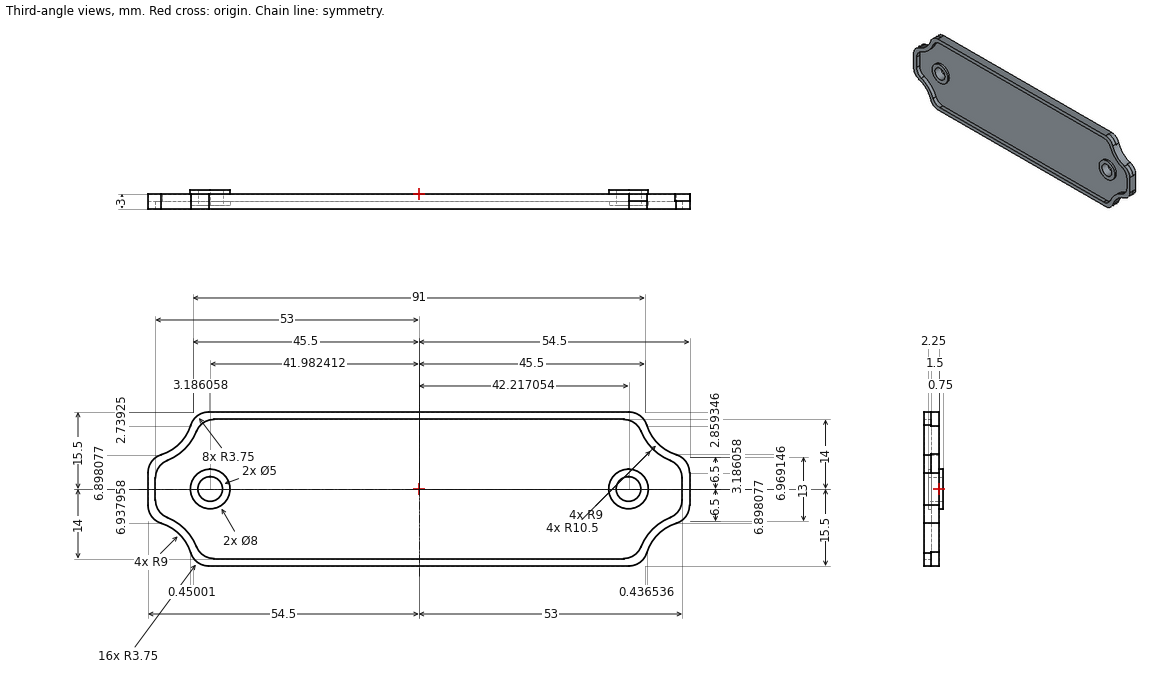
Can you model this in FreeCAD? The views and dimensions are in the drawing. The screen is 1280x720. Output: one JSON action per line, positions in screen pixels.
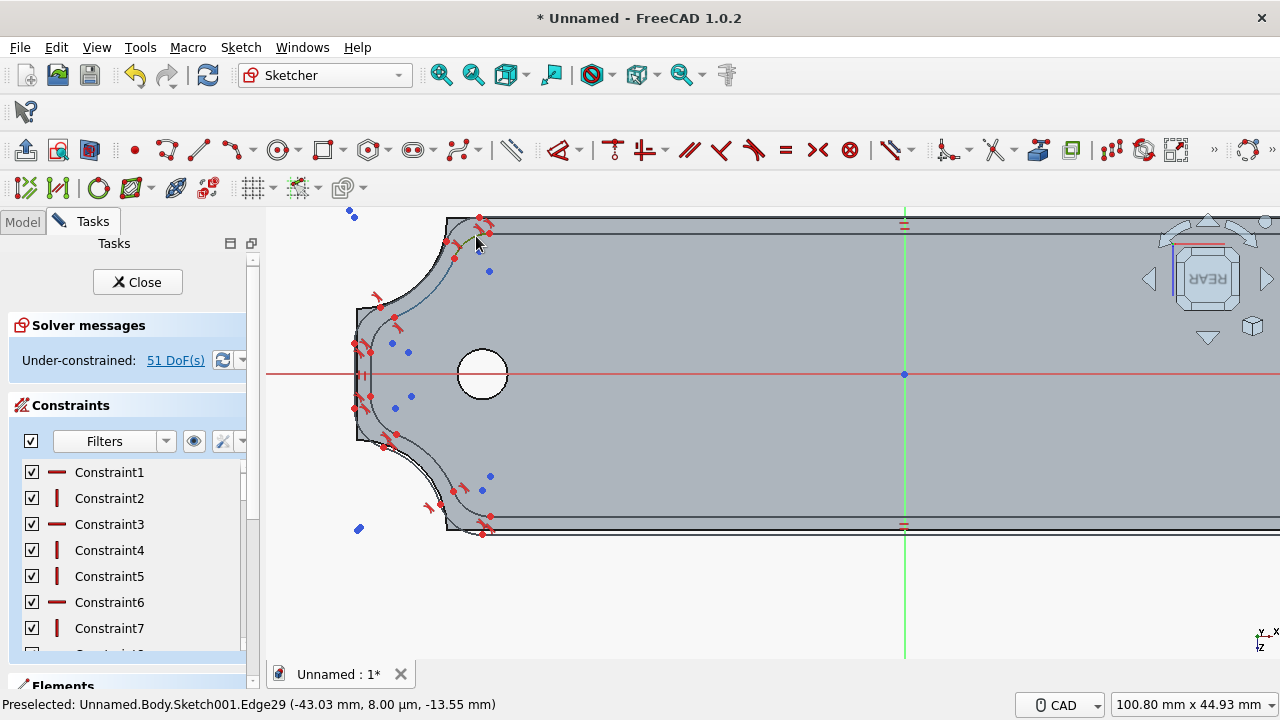
{"action": "left_click", "coordinate": [754, 150]}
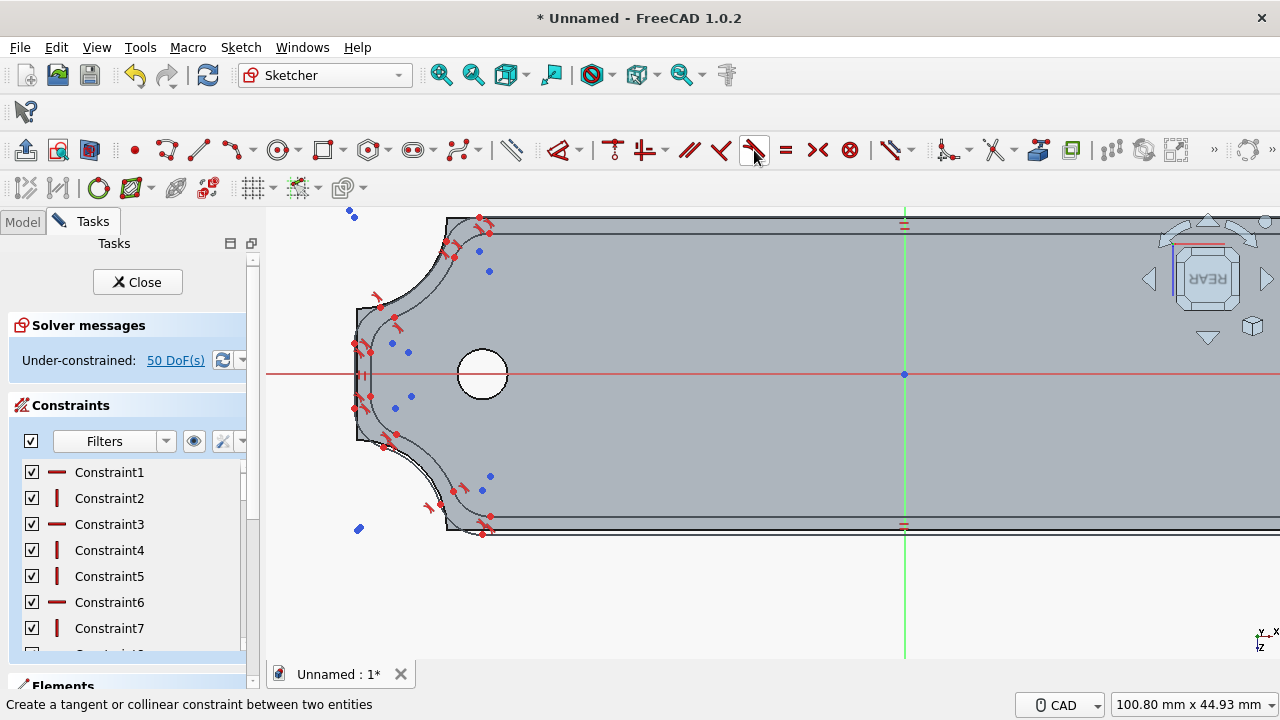
{"action": "scroll", "coordinate": [461, 504], "scroll_direction": "down", "scroll_amount": 3}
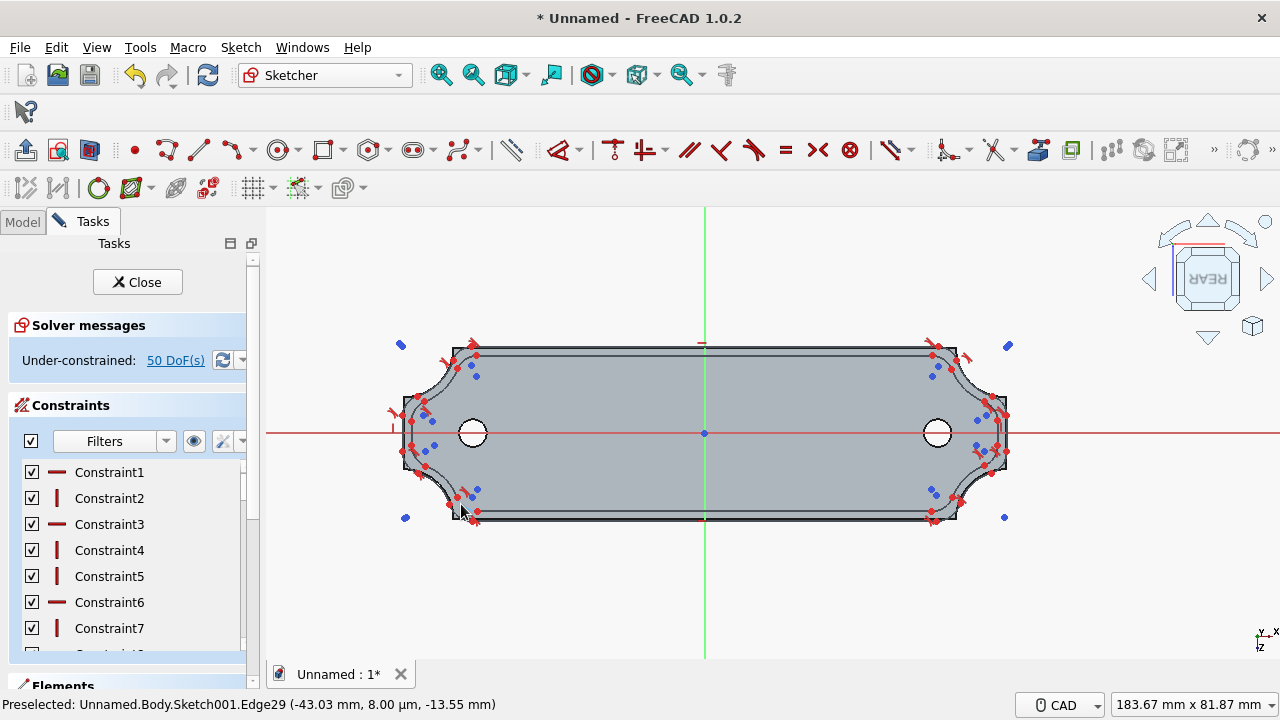
{"action": "scroll", "coordinate": [948, 363], "scroll_direction": "up", "scroll_amount": 4}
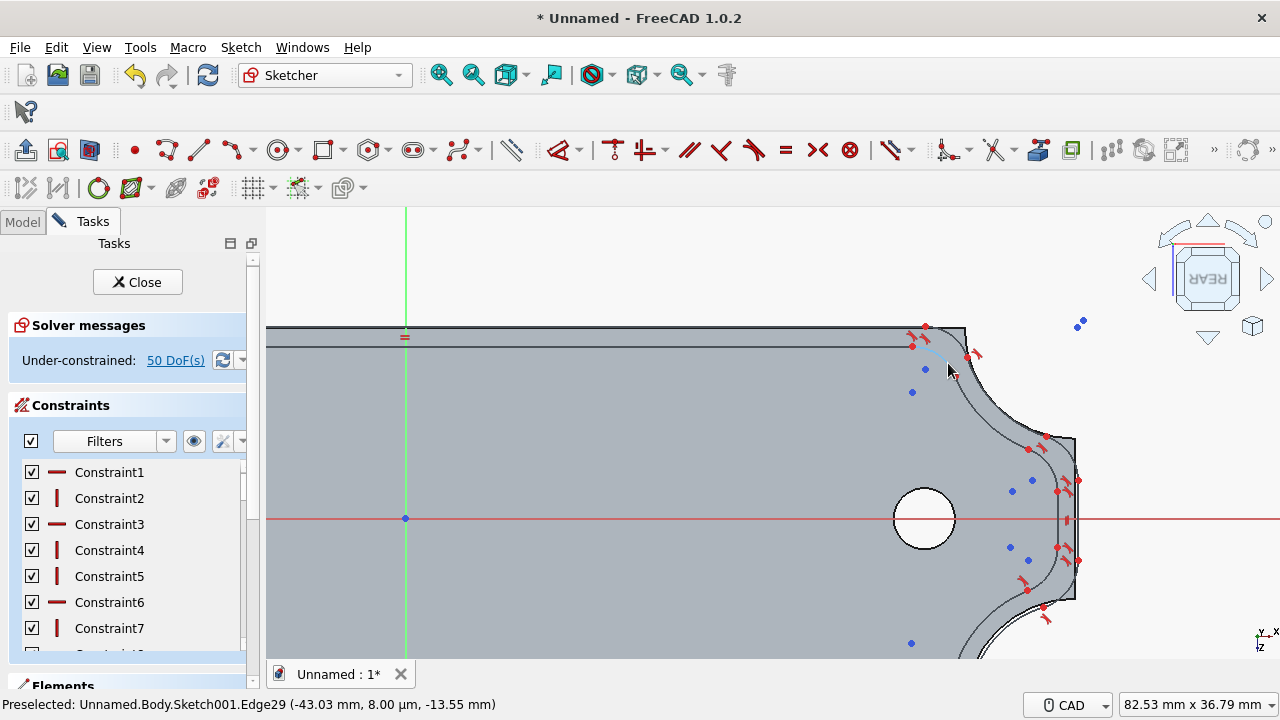
{"action": "left_click", "coordinate": [947, 362]}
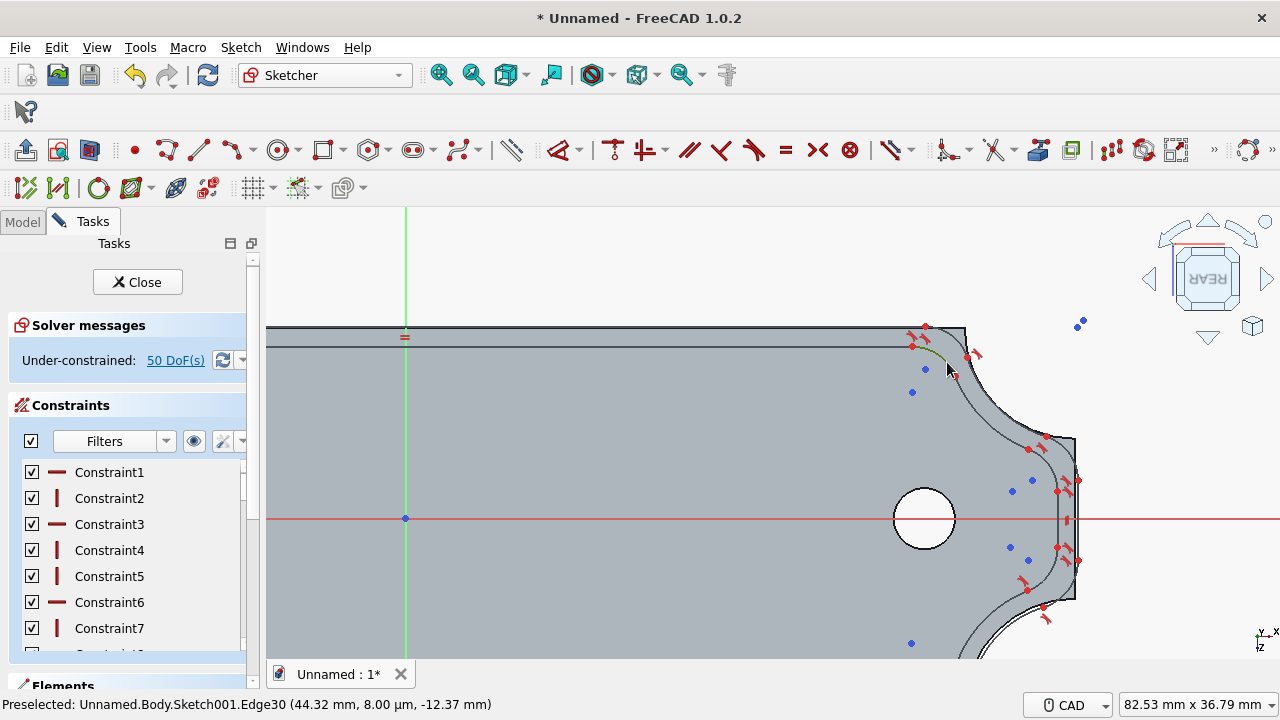
{"action": "left_click", "coordinate": [971, 404]}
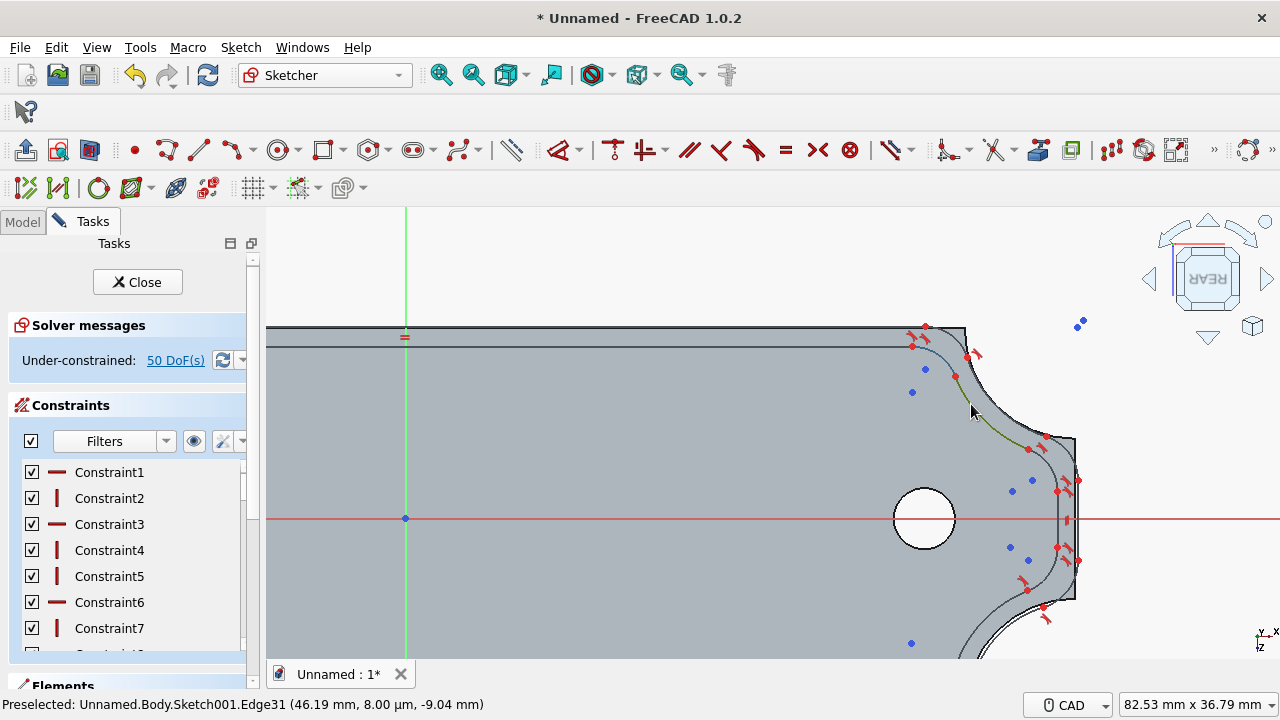
{"action": "left_click", "coordinate": [754, 150]}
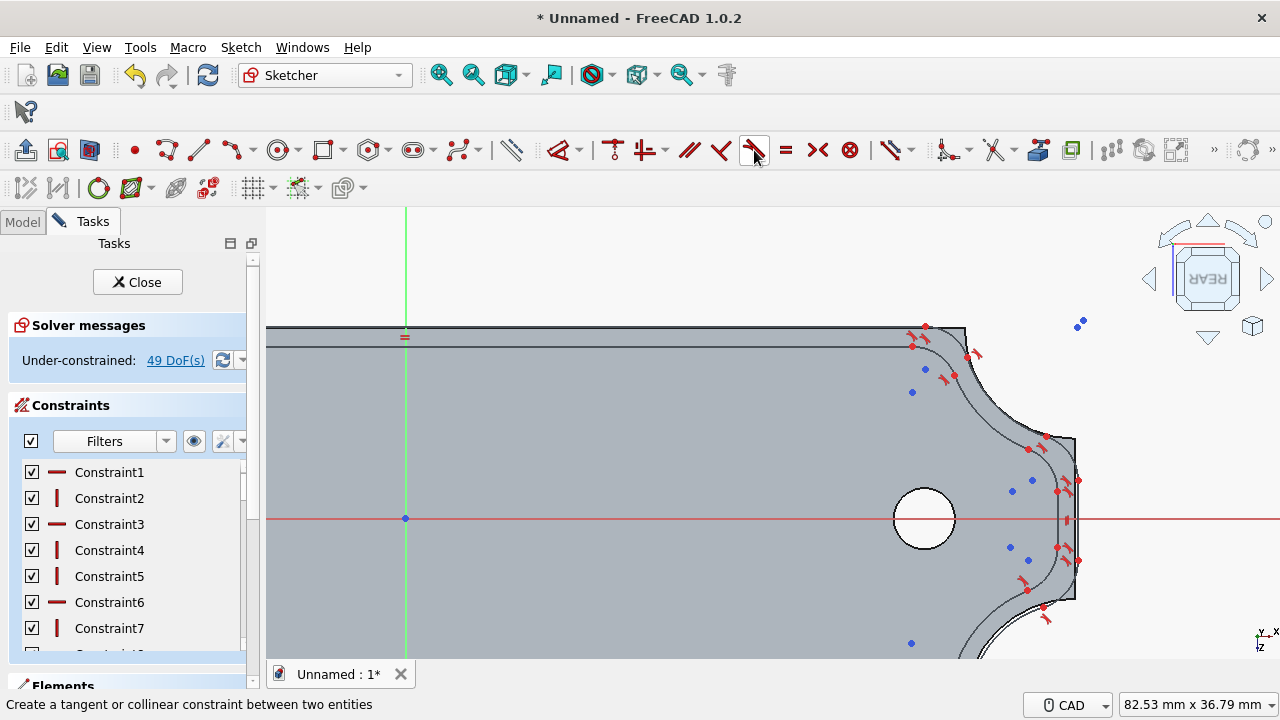
{"action": "left_click", "coordinate": [970, 404]}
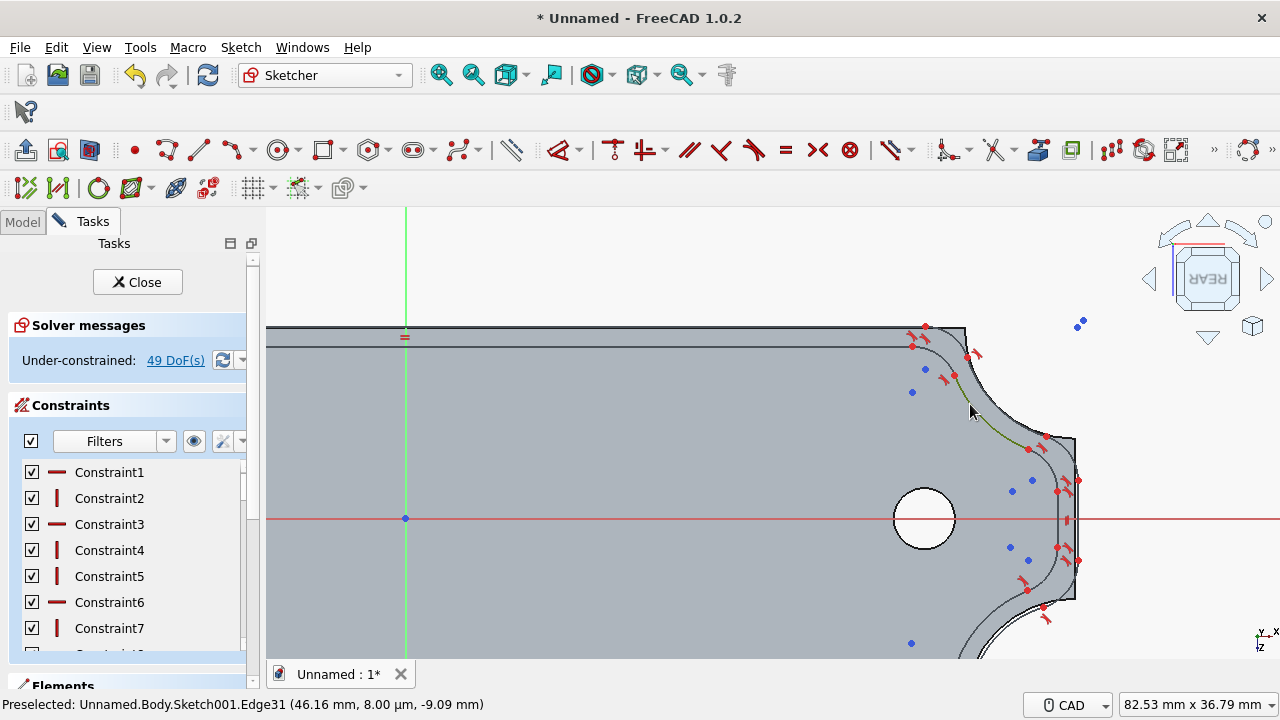
{"action": "left_click", "coordinate": [1055, 476]}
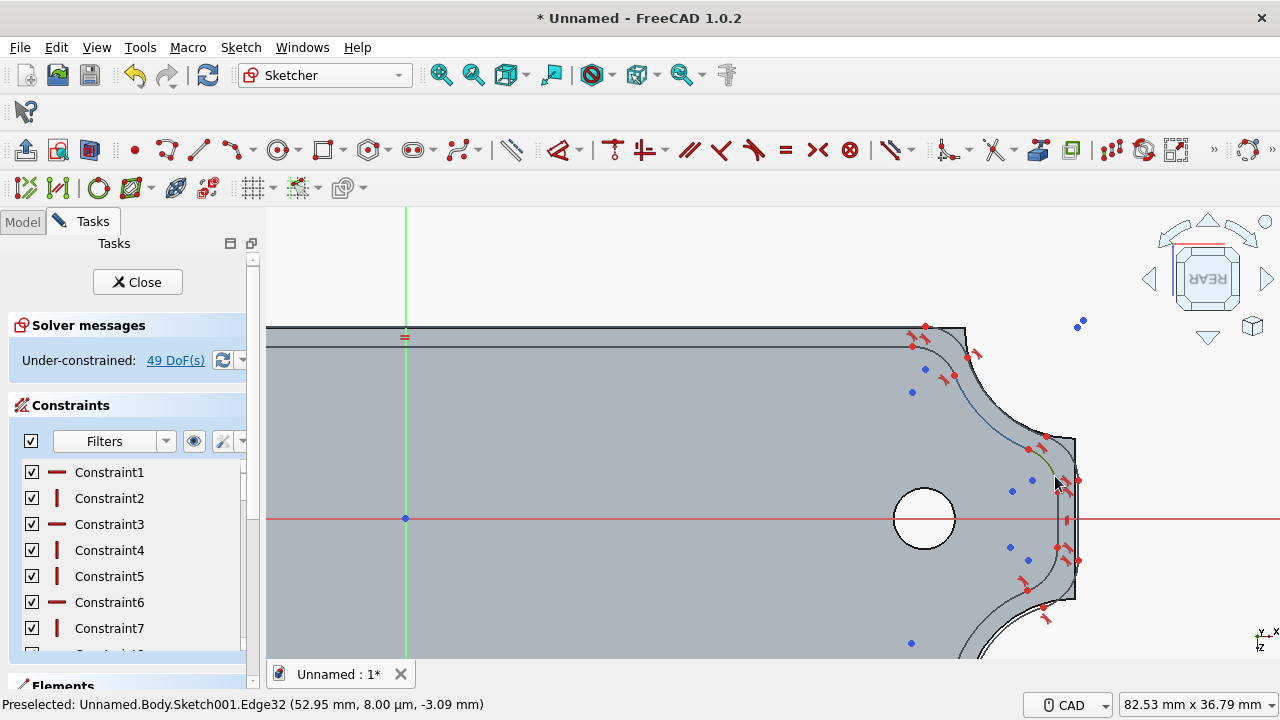
{"action": "left_click", "coordinate": [754, 150]}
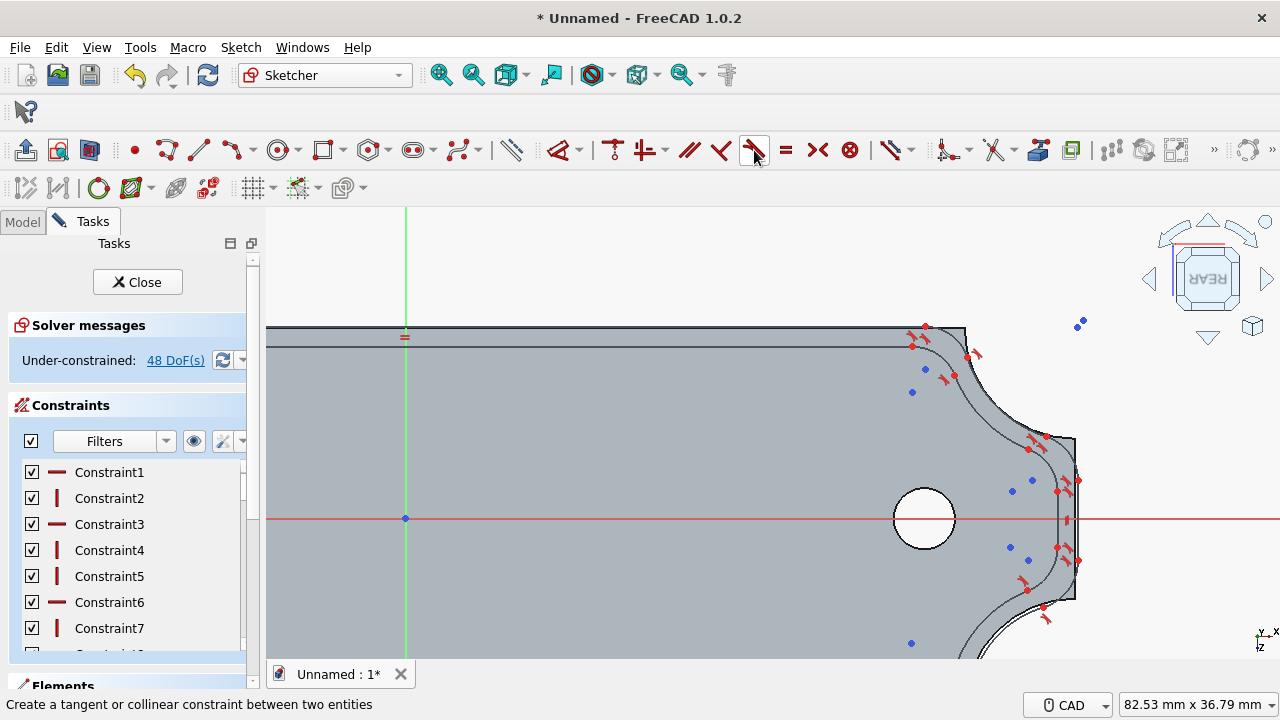
{"action": "left_click", "coordinate": [1016, 620]}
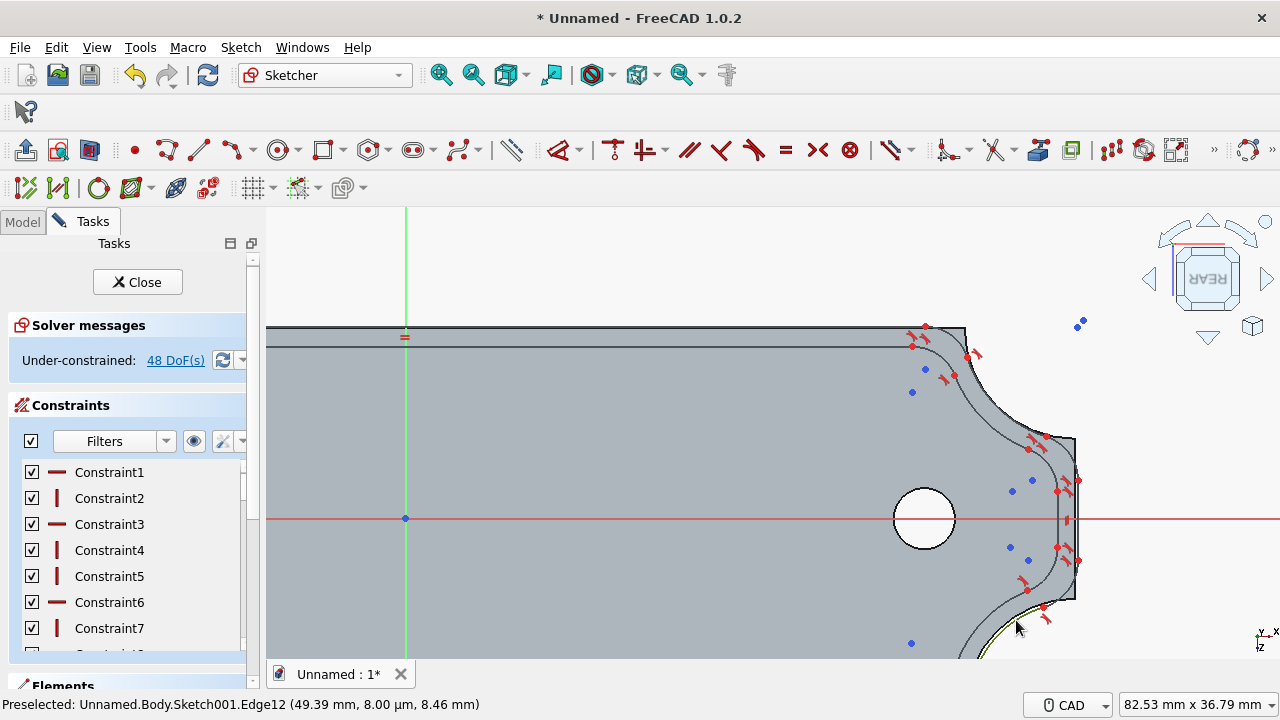
{"action": "left_click", "coordinate": [1001, 606]}